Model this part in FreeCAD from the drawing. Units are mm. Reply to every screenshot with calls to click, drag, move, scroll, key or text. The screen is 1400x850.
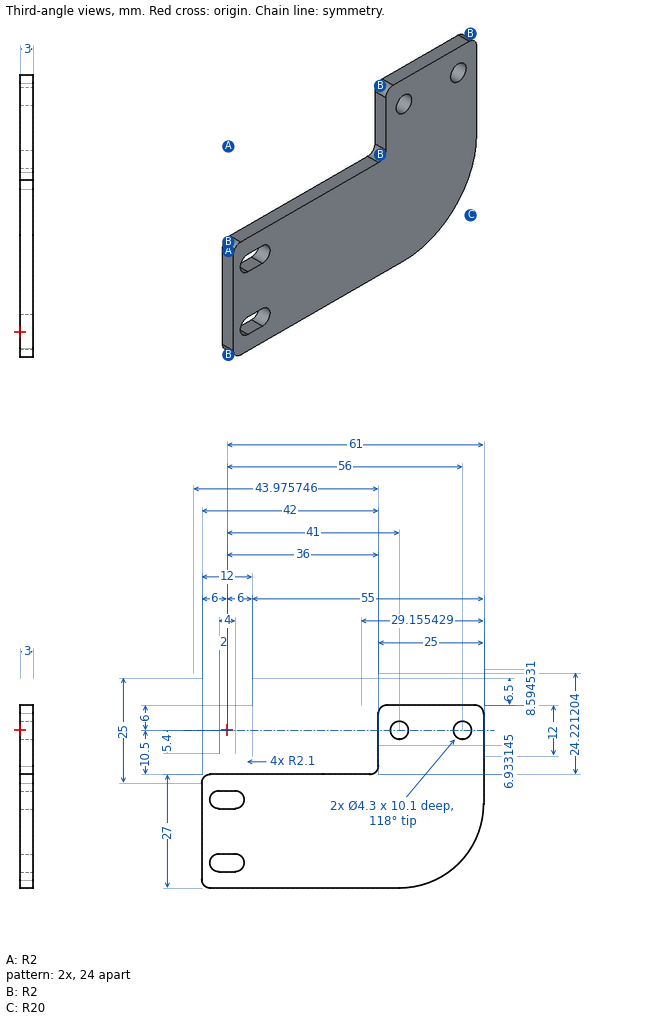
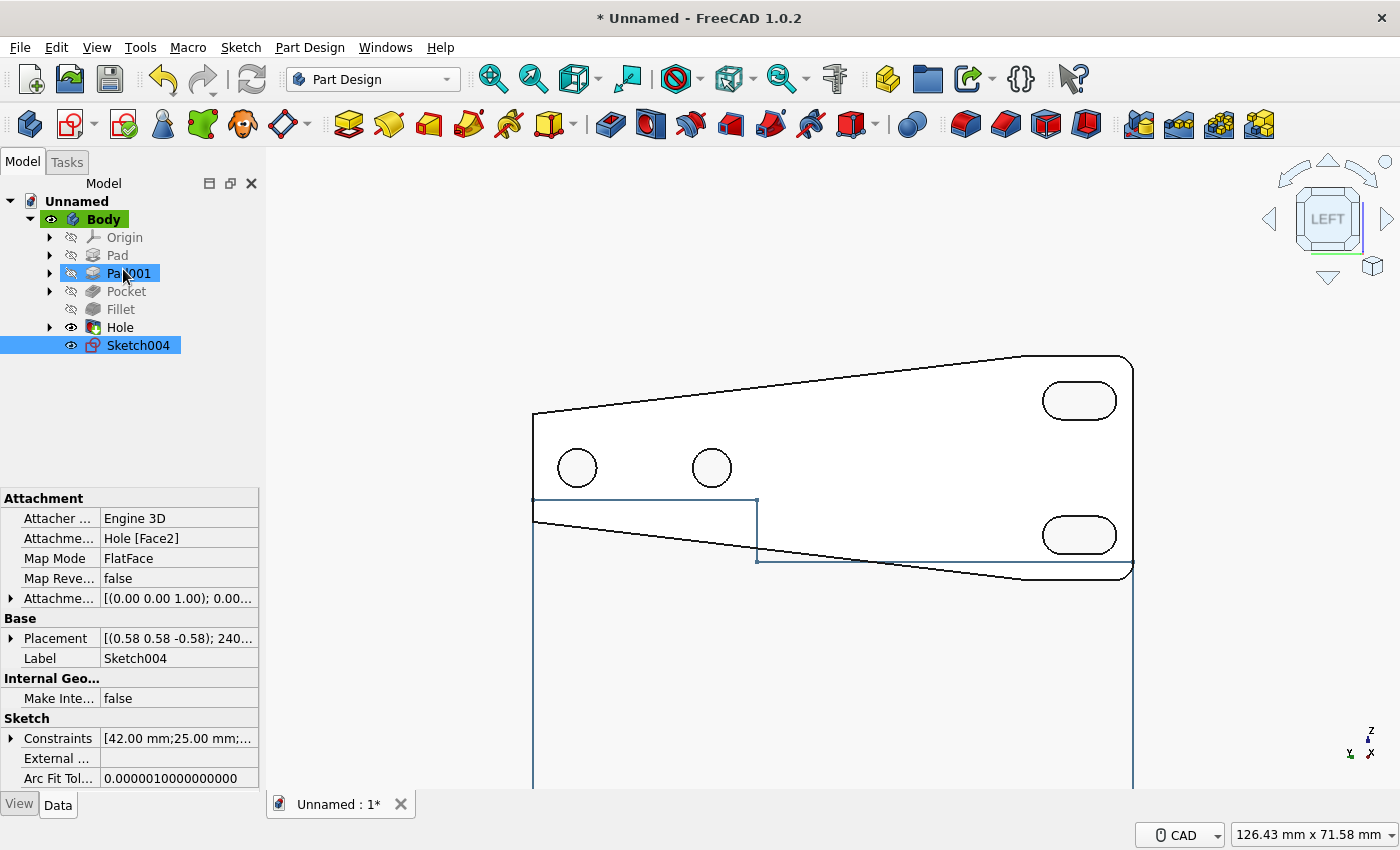
click(350, 124)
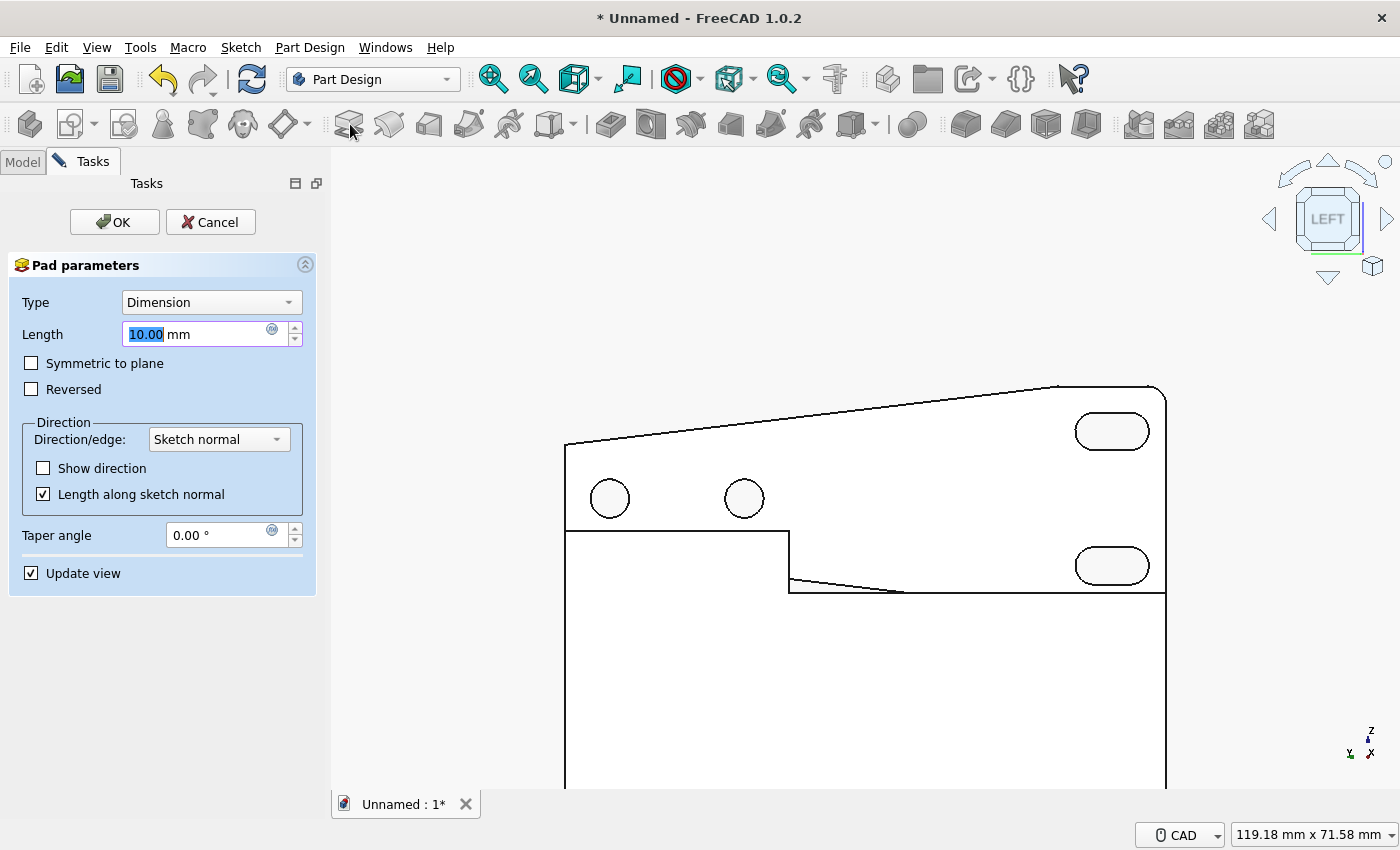
text(3)
key(Tab)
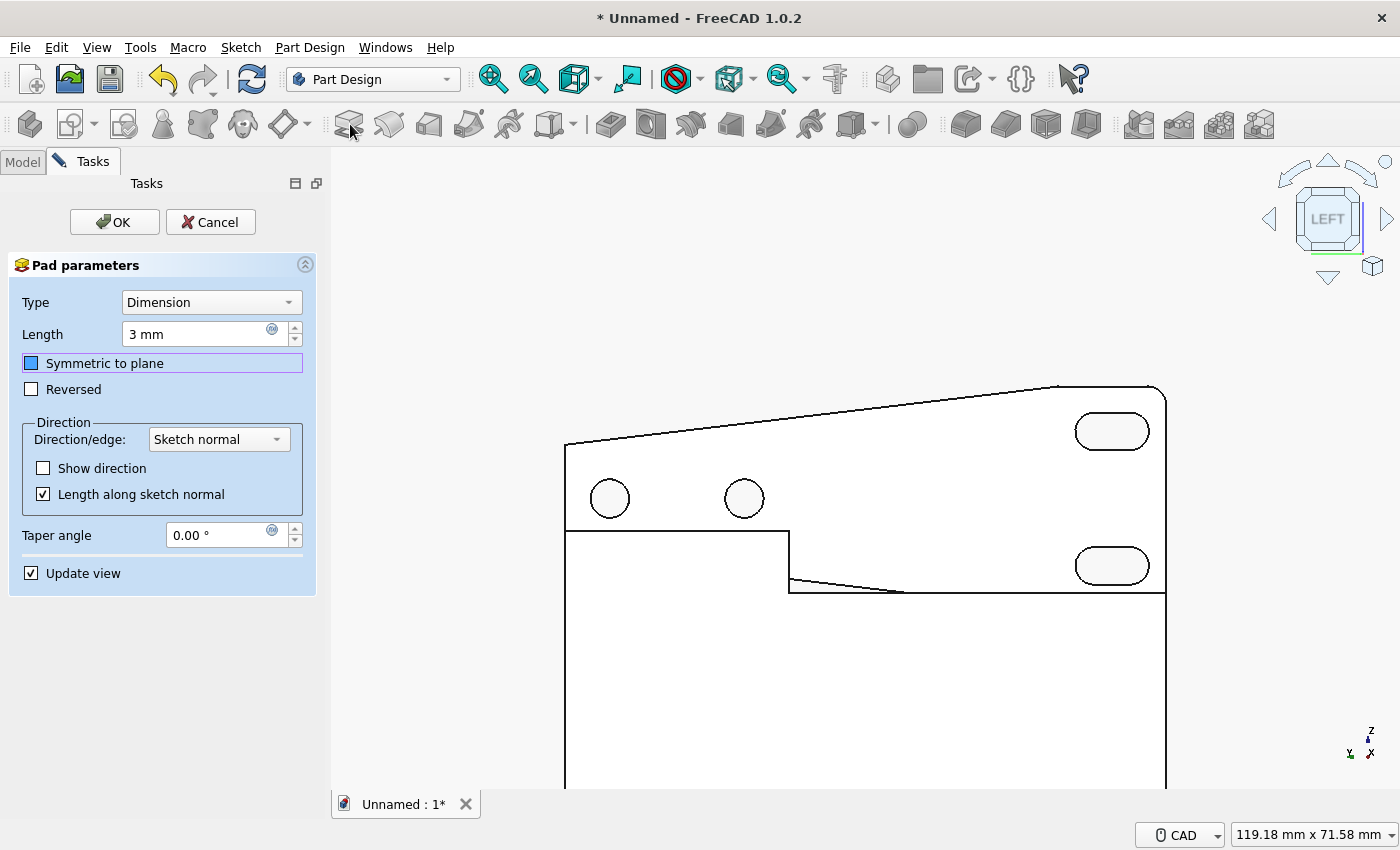
click(30, 389)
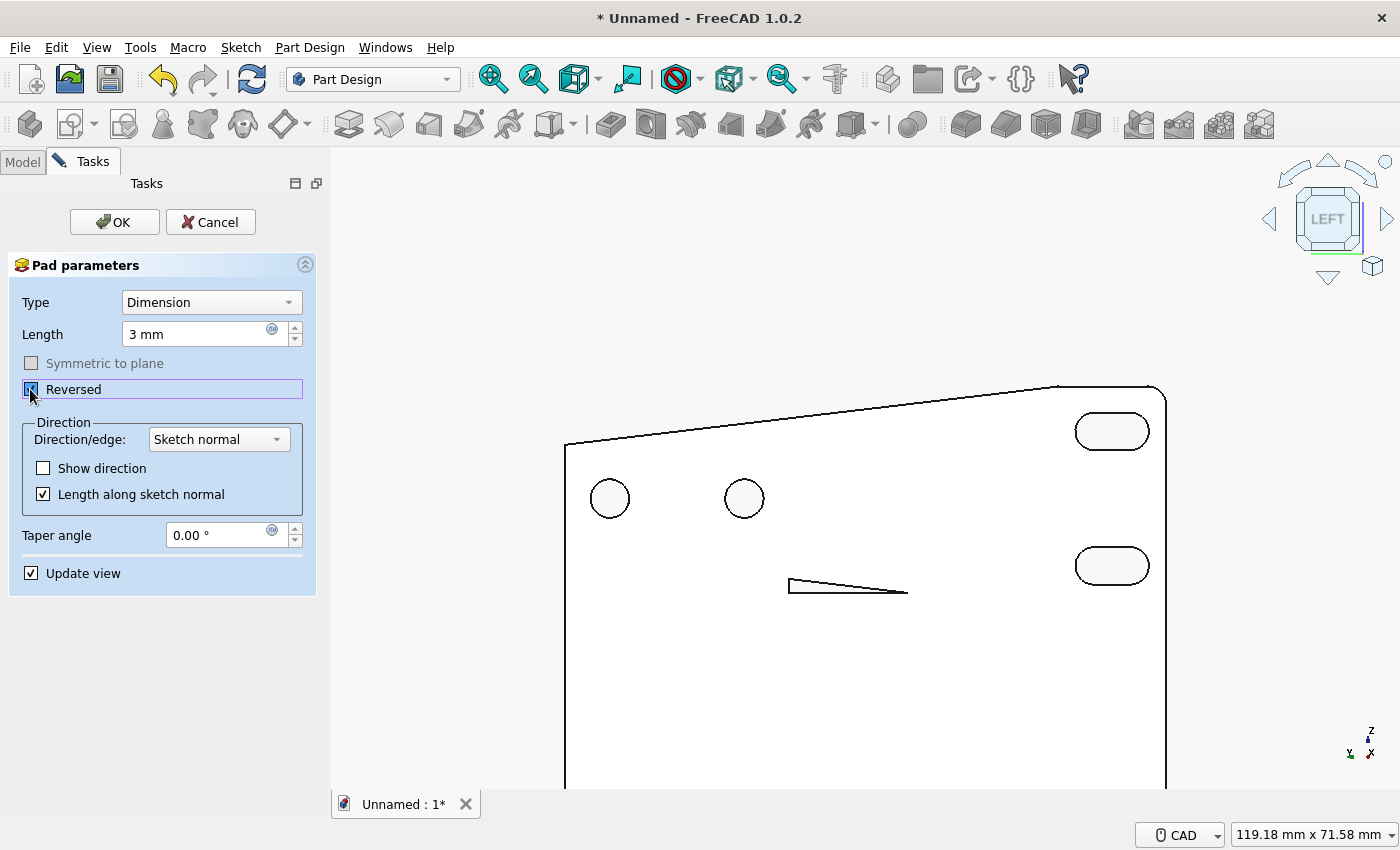
click(115, 222)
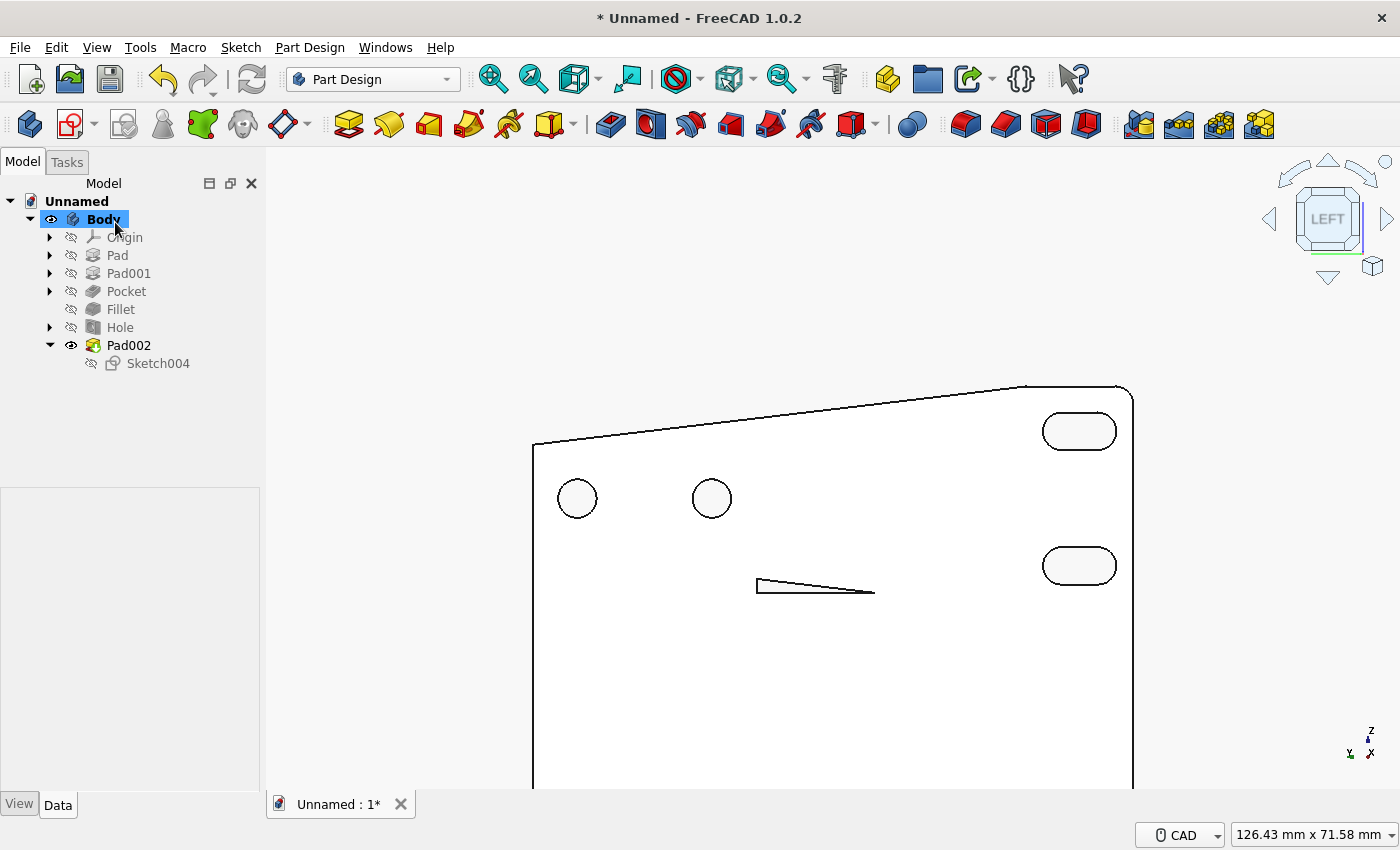
click(494, 80)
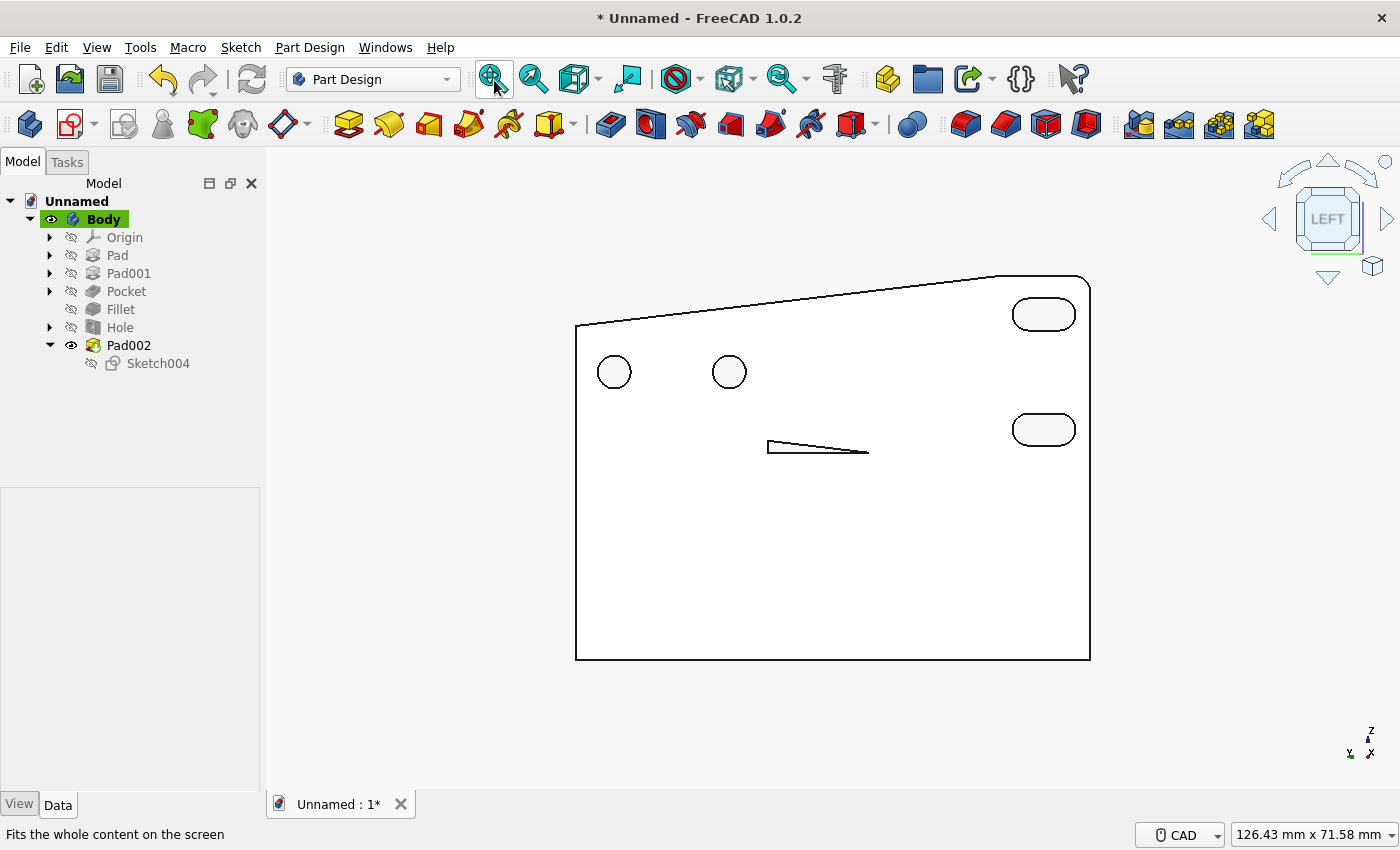
click(116, 291)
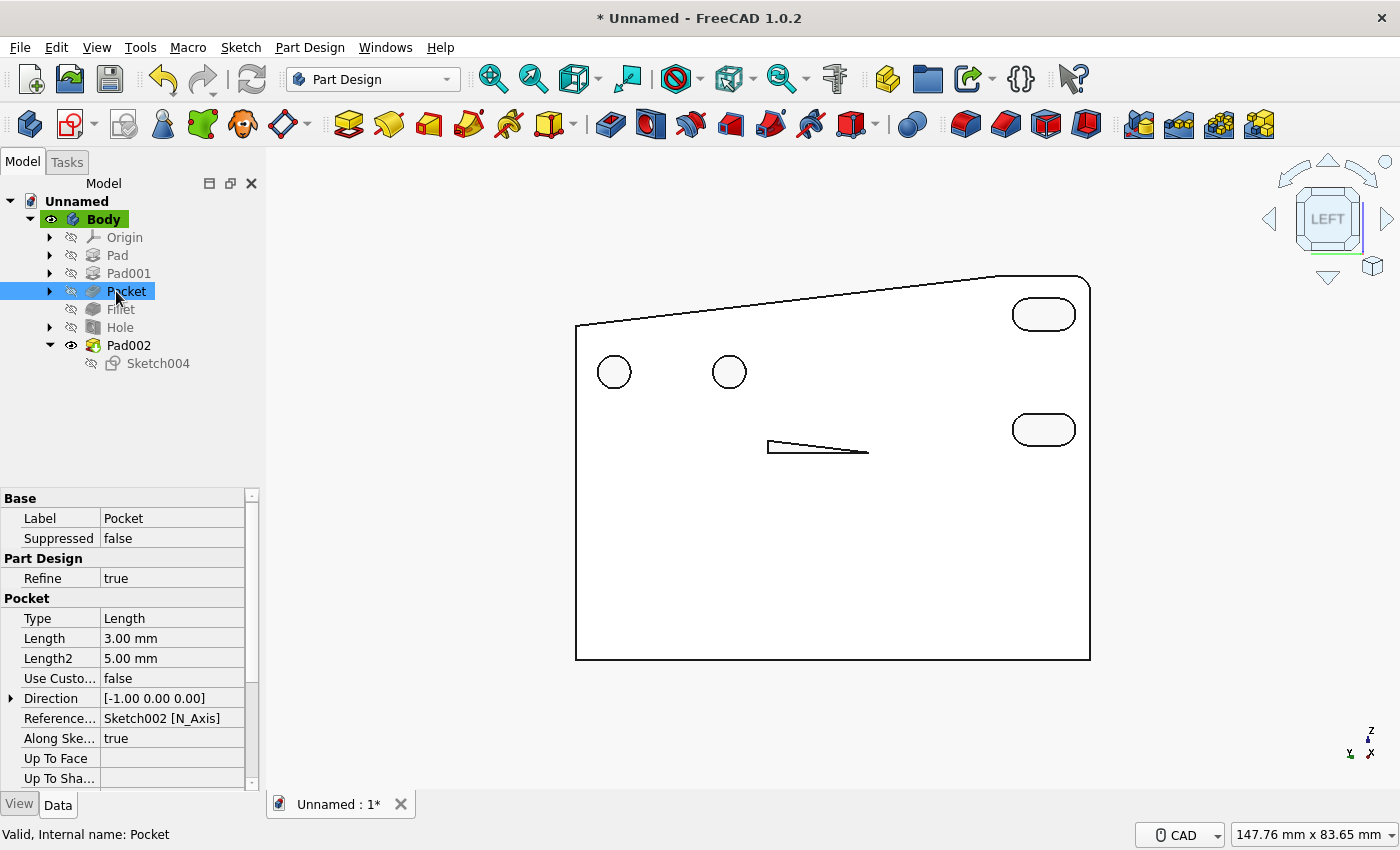
click(1180, 124)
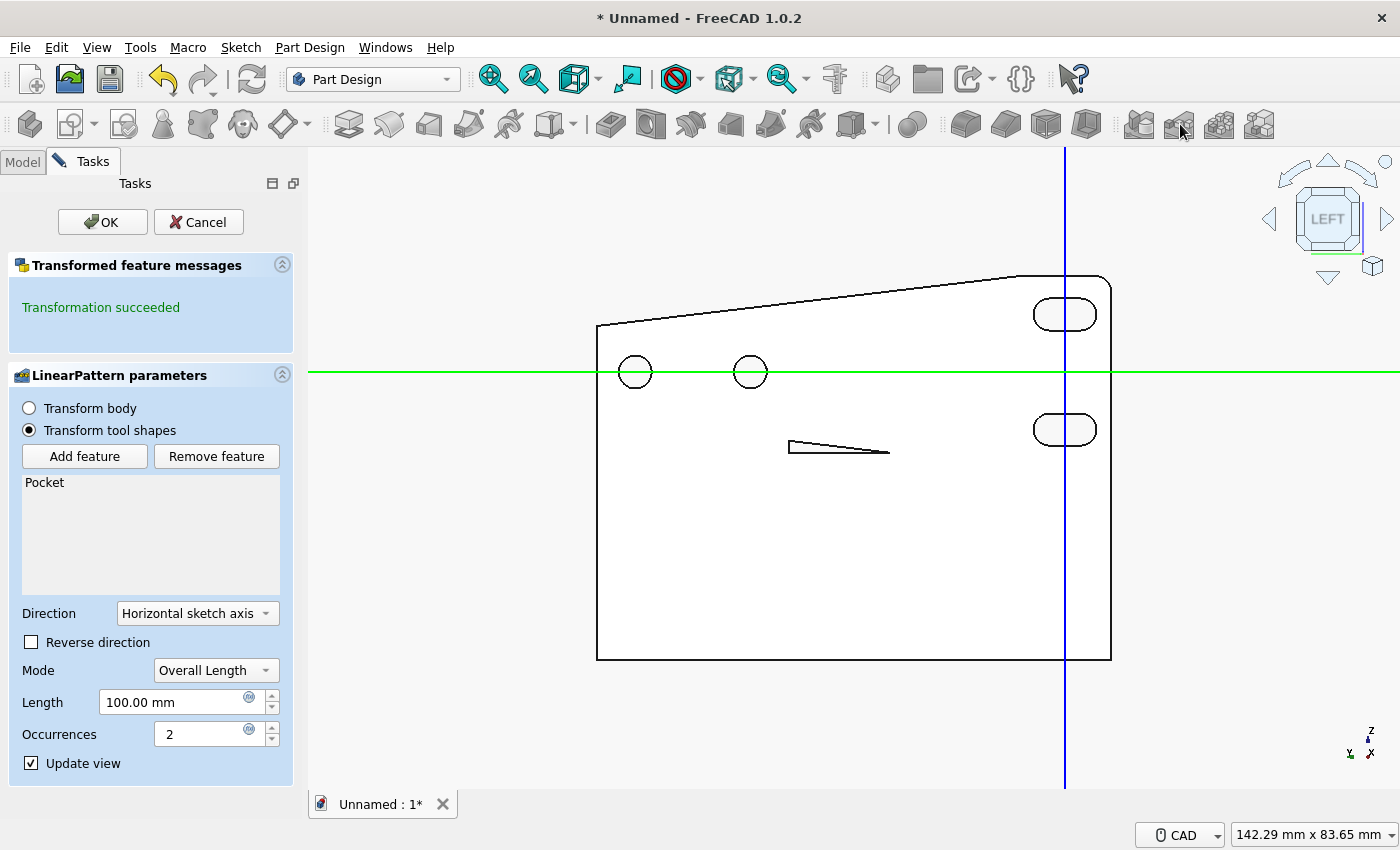
click(198, 614)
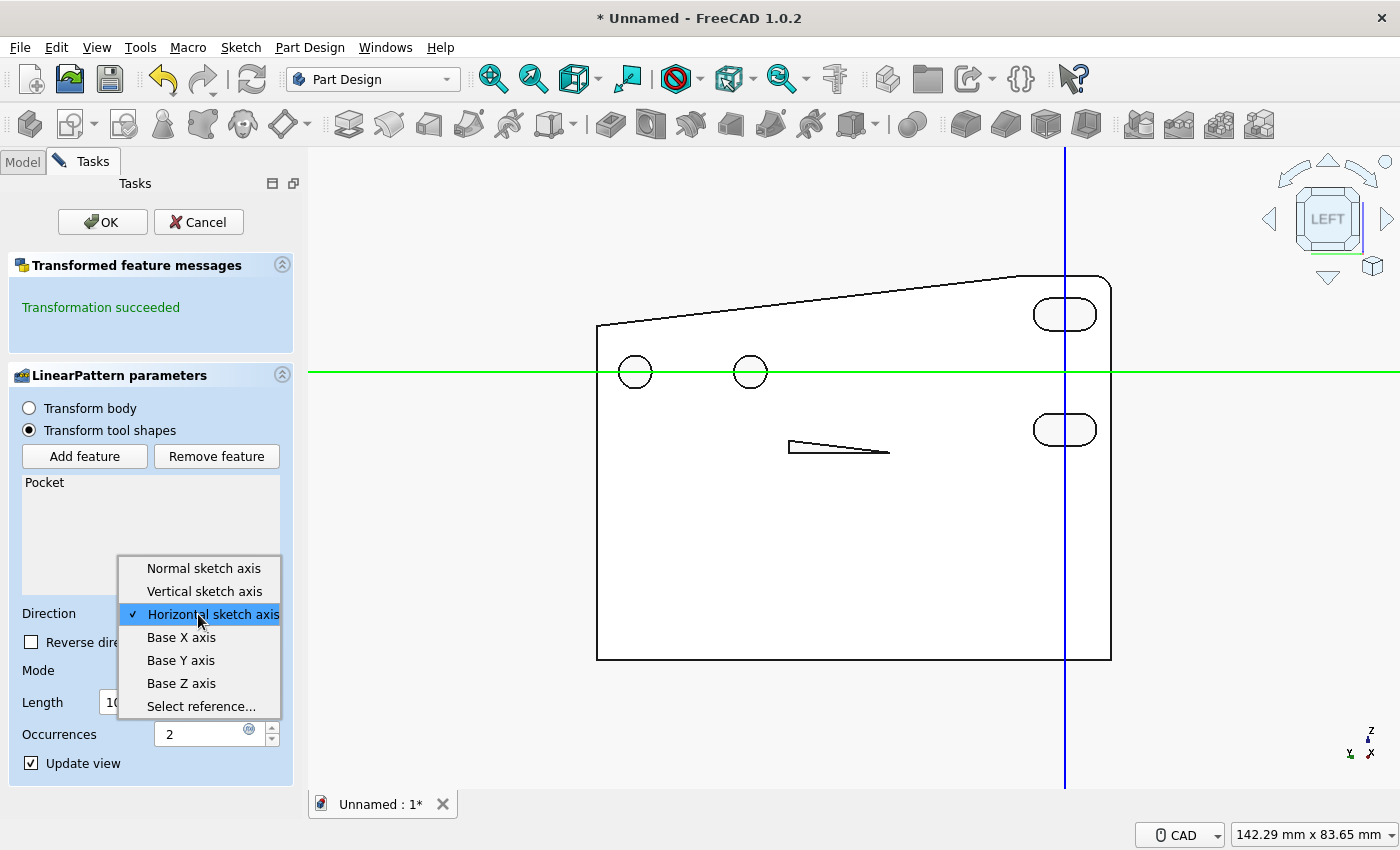
click(198, 684)